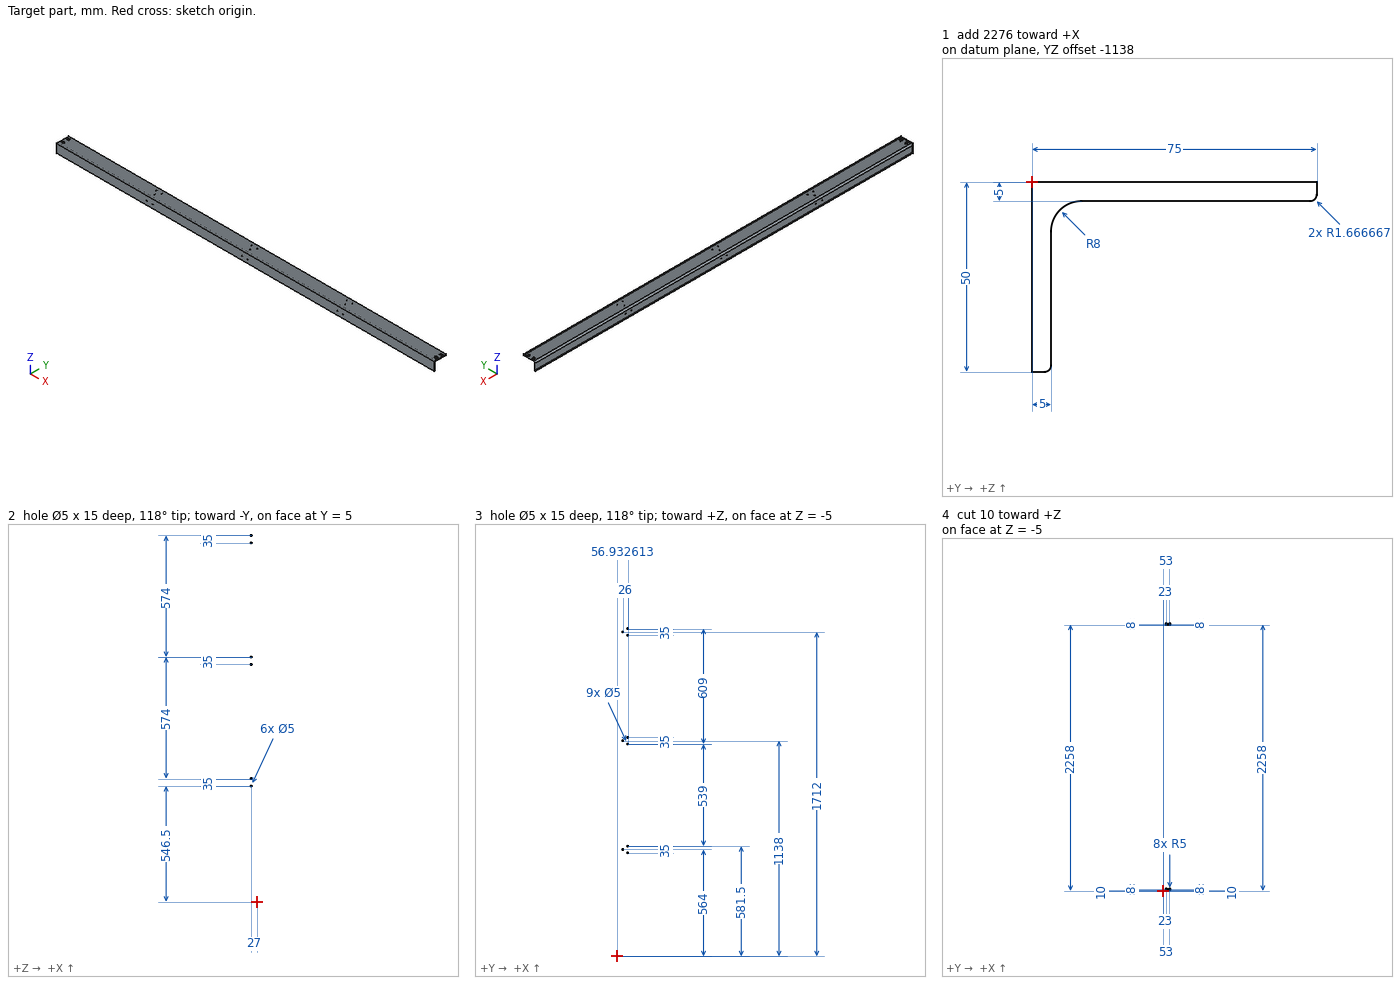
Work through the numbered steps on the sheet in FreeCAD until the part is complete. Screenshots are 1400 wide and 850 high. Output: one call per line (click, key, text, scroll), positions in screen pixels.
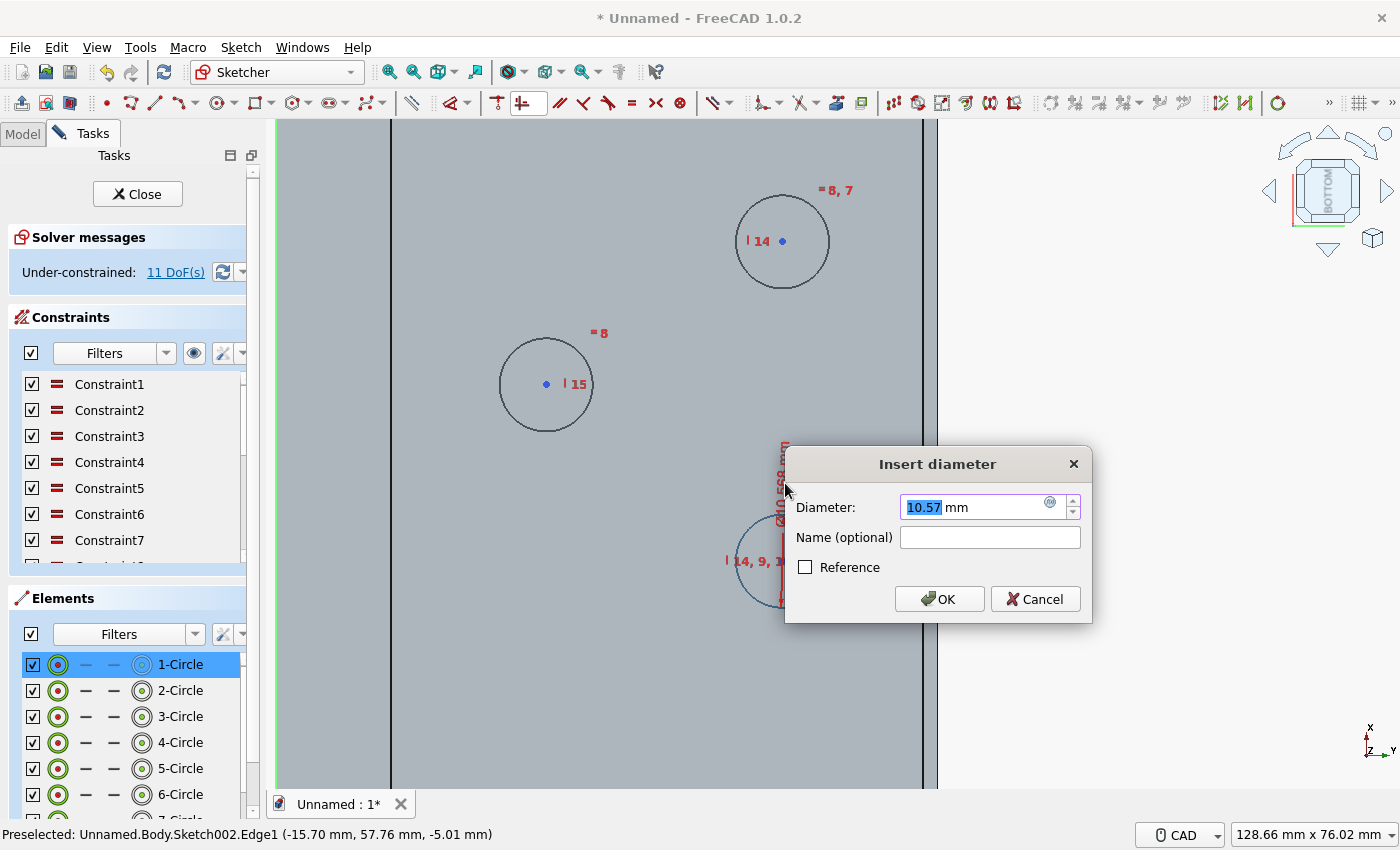
text(5)
key(Return)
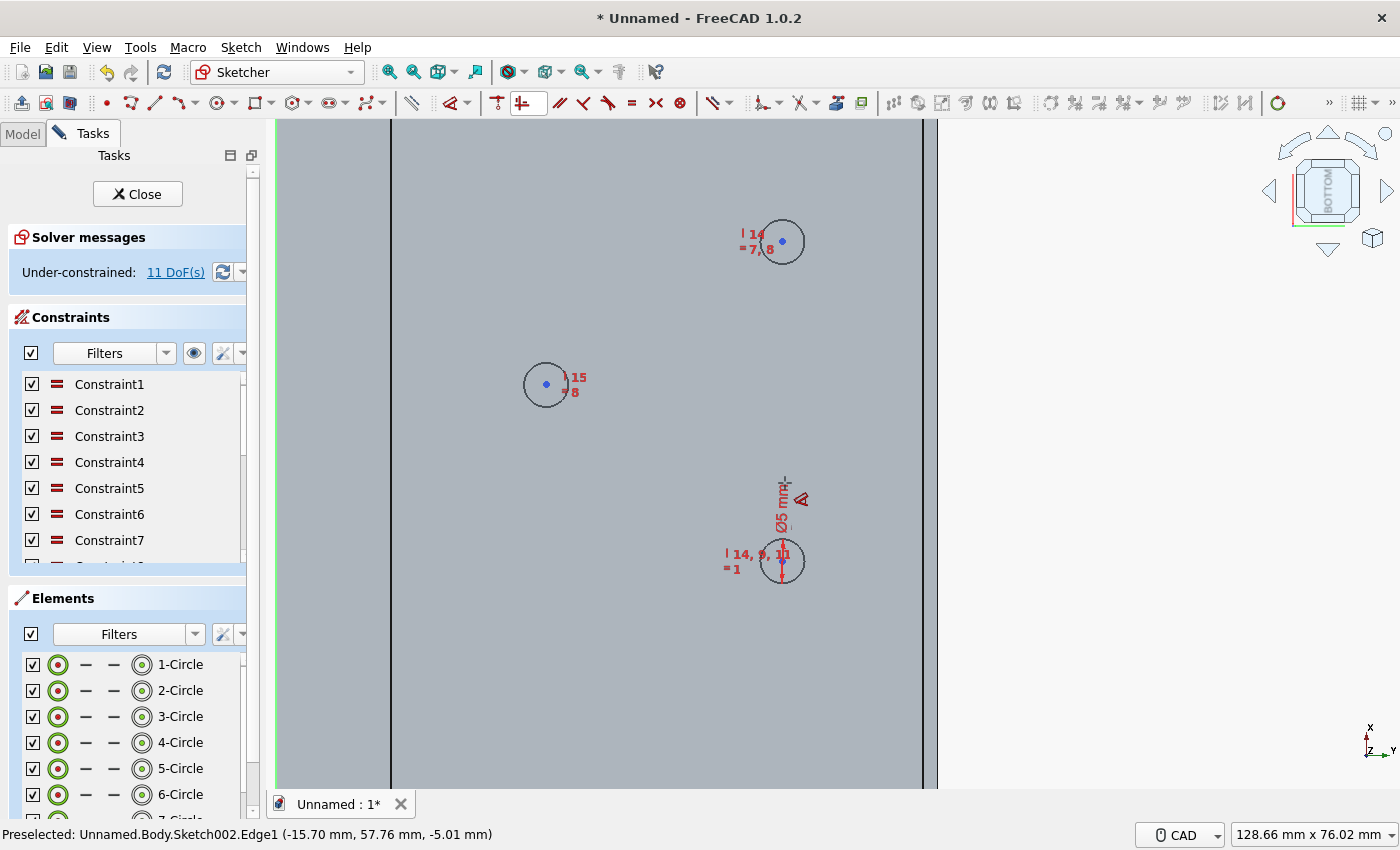
scroll(772, 374, down, 17)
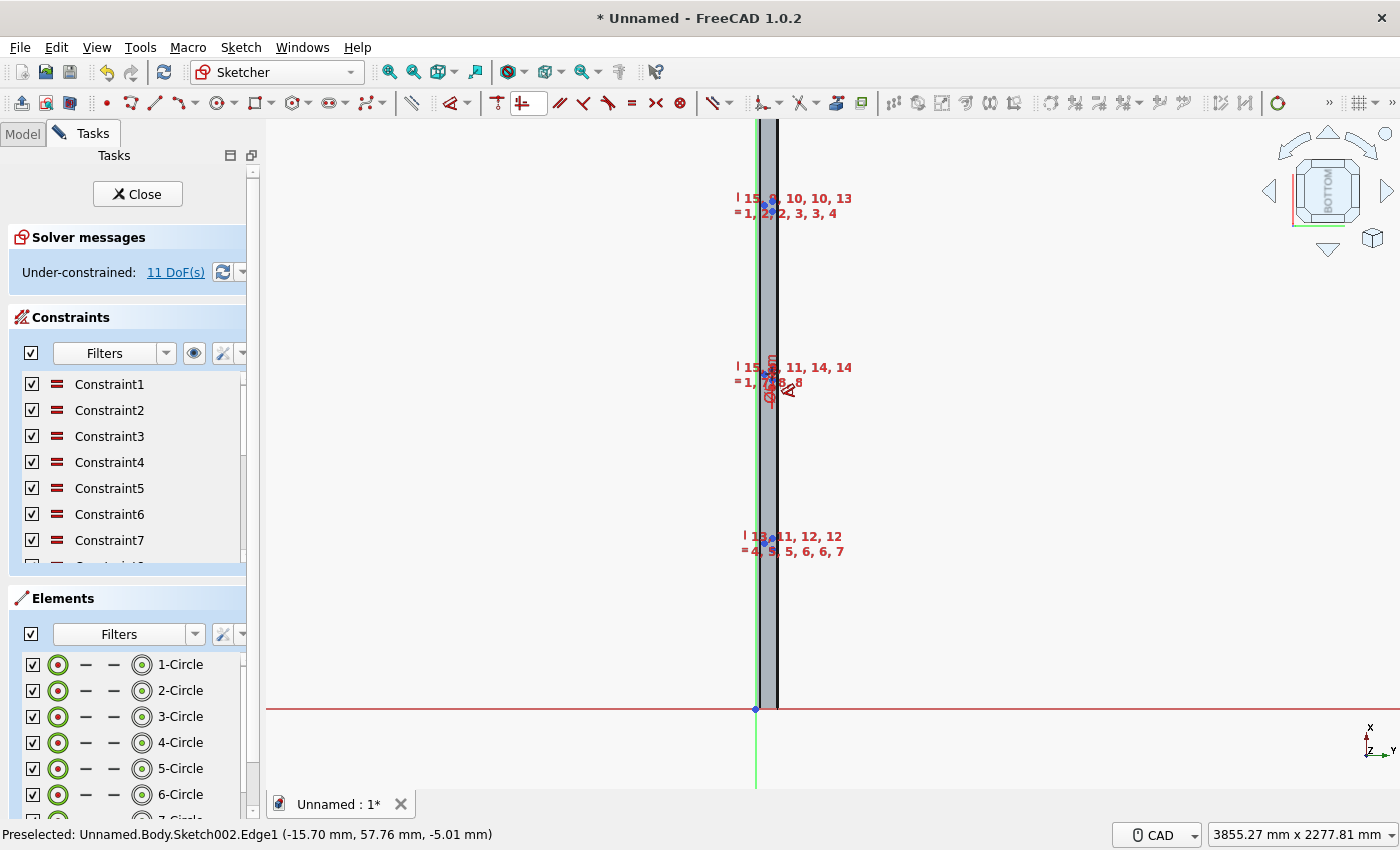
scroll(765, 544, up, 2)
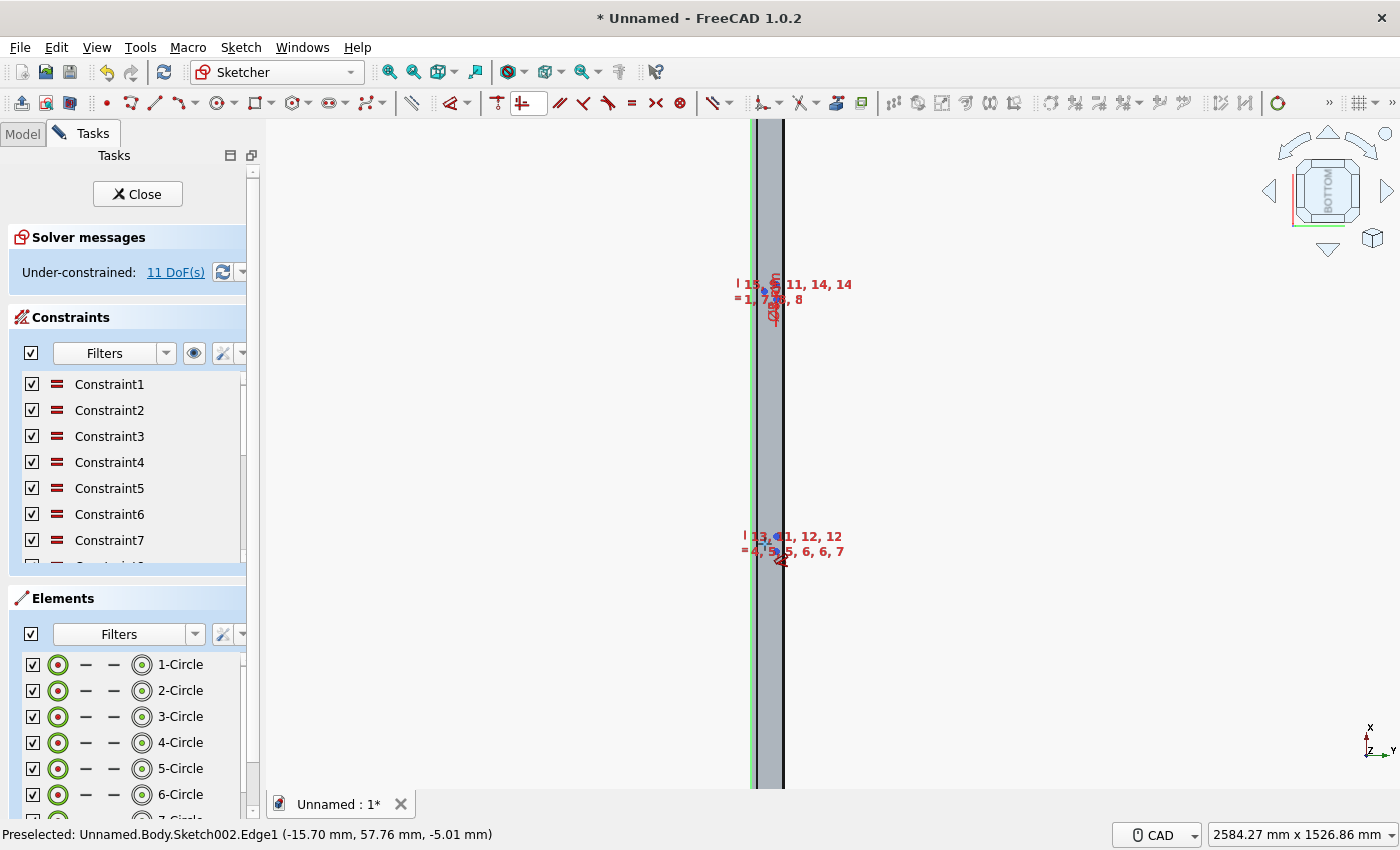
click(765, 544)
click(717, 652)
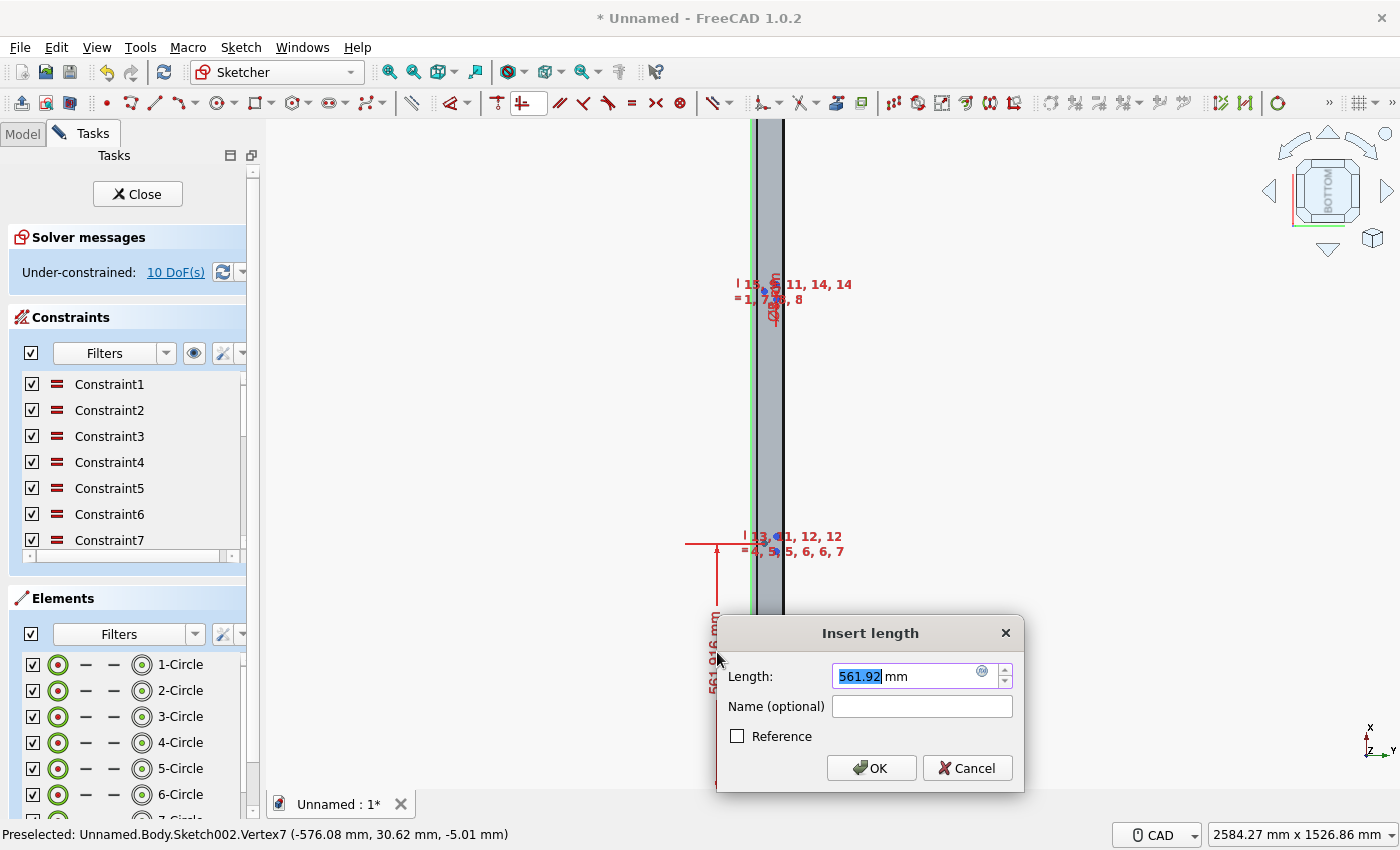
text(564)
key(Return)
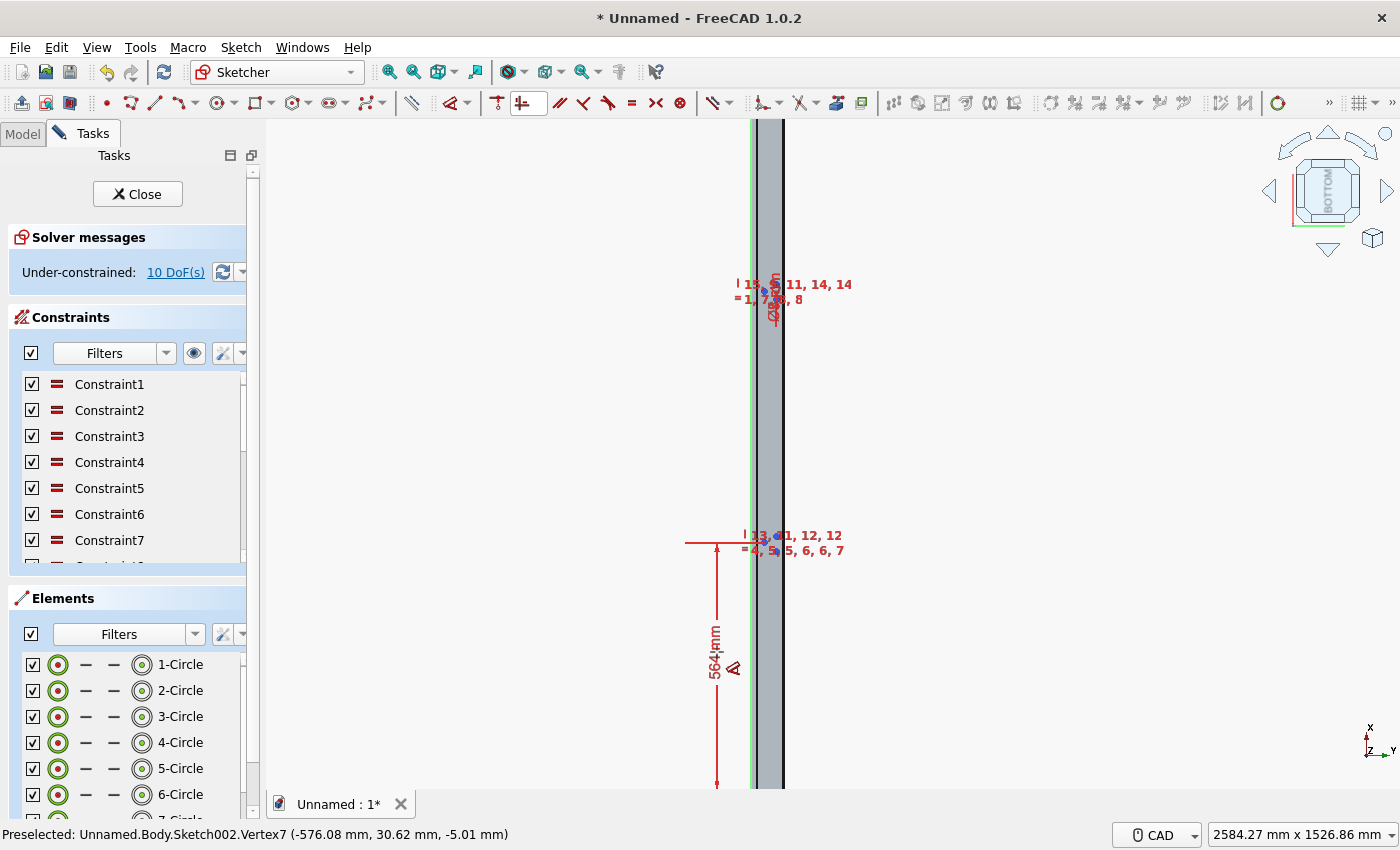
scroll(765, 507, down, 3)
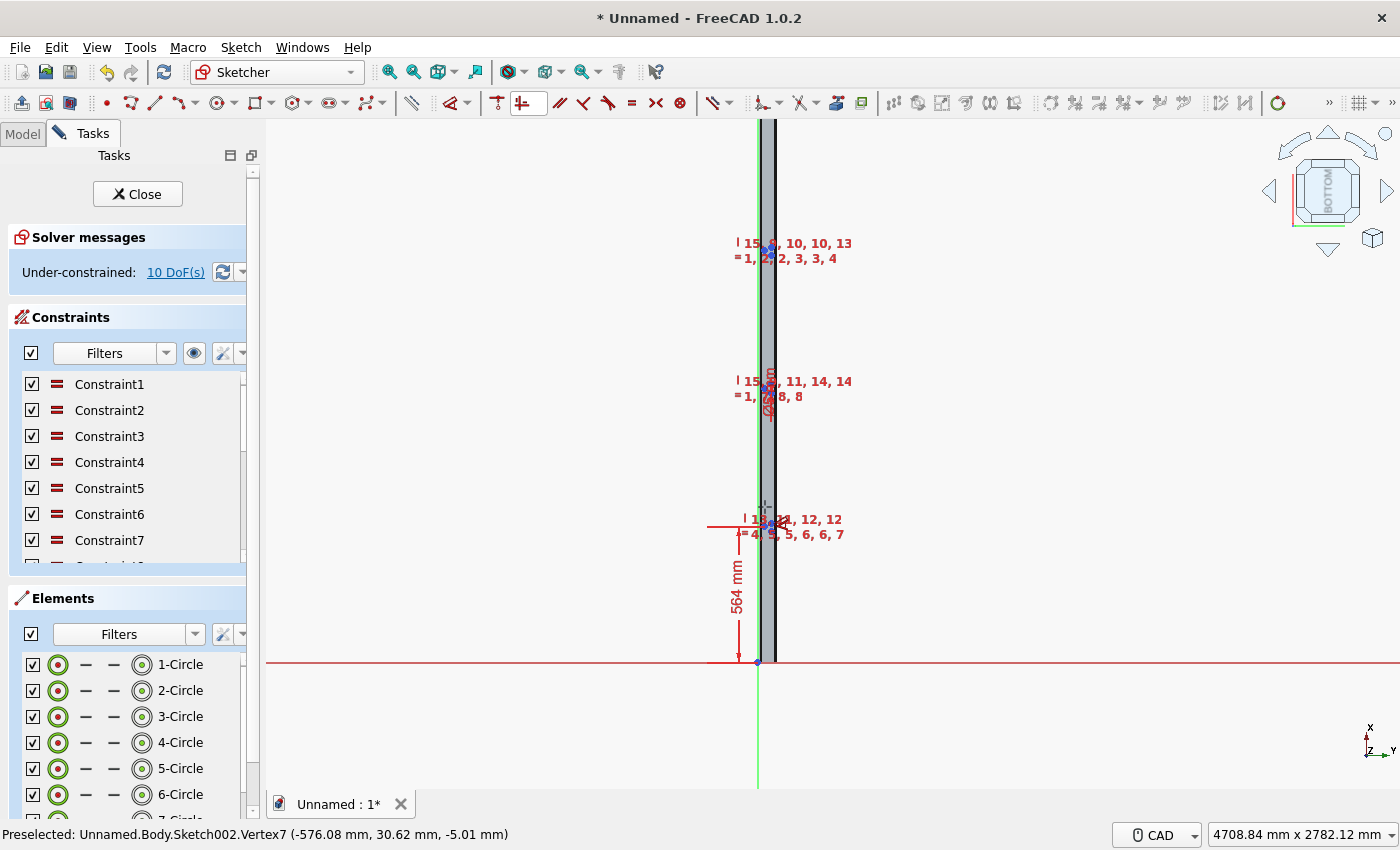
scroll(771, 247, up, 8)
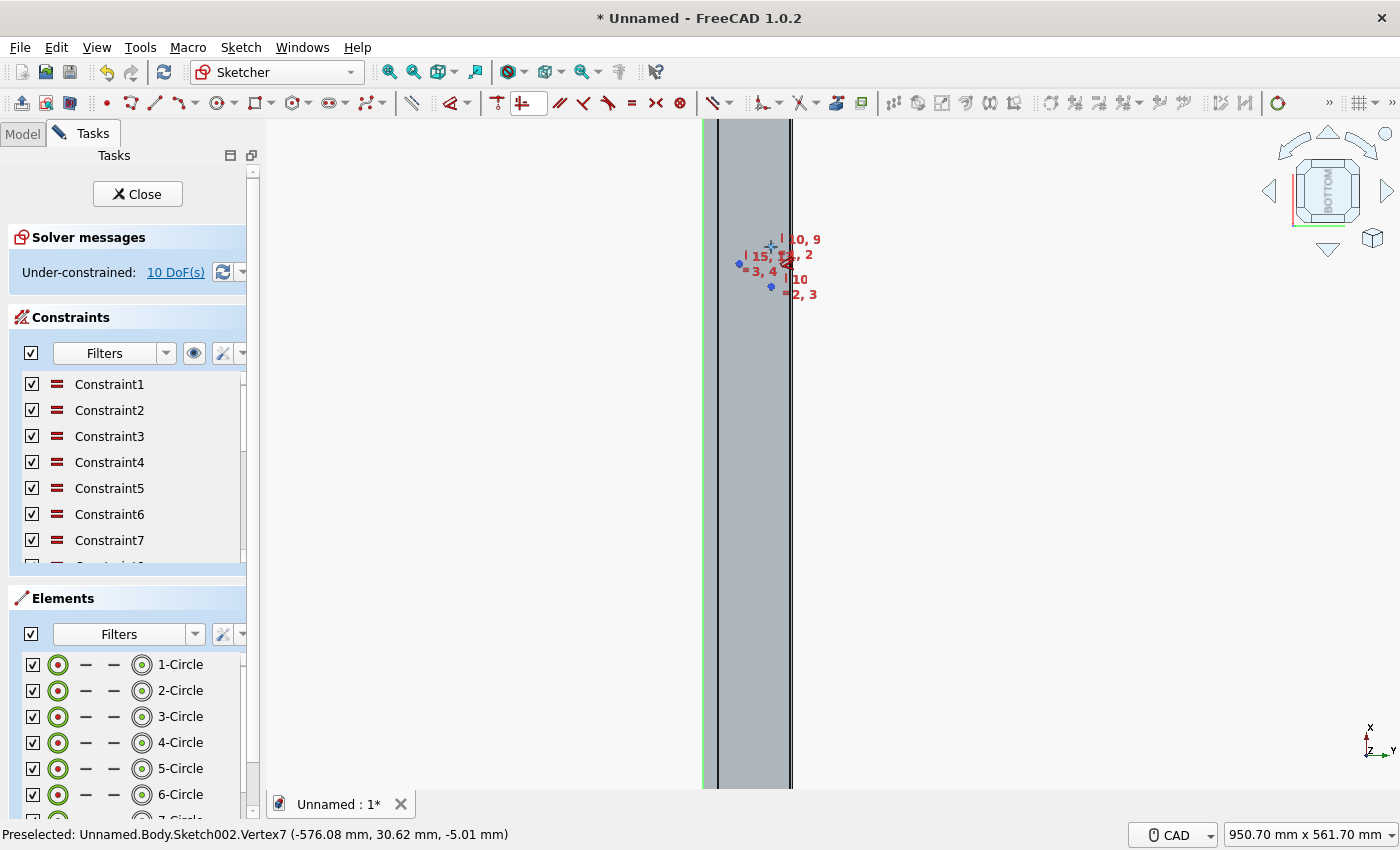
click(771, 247)